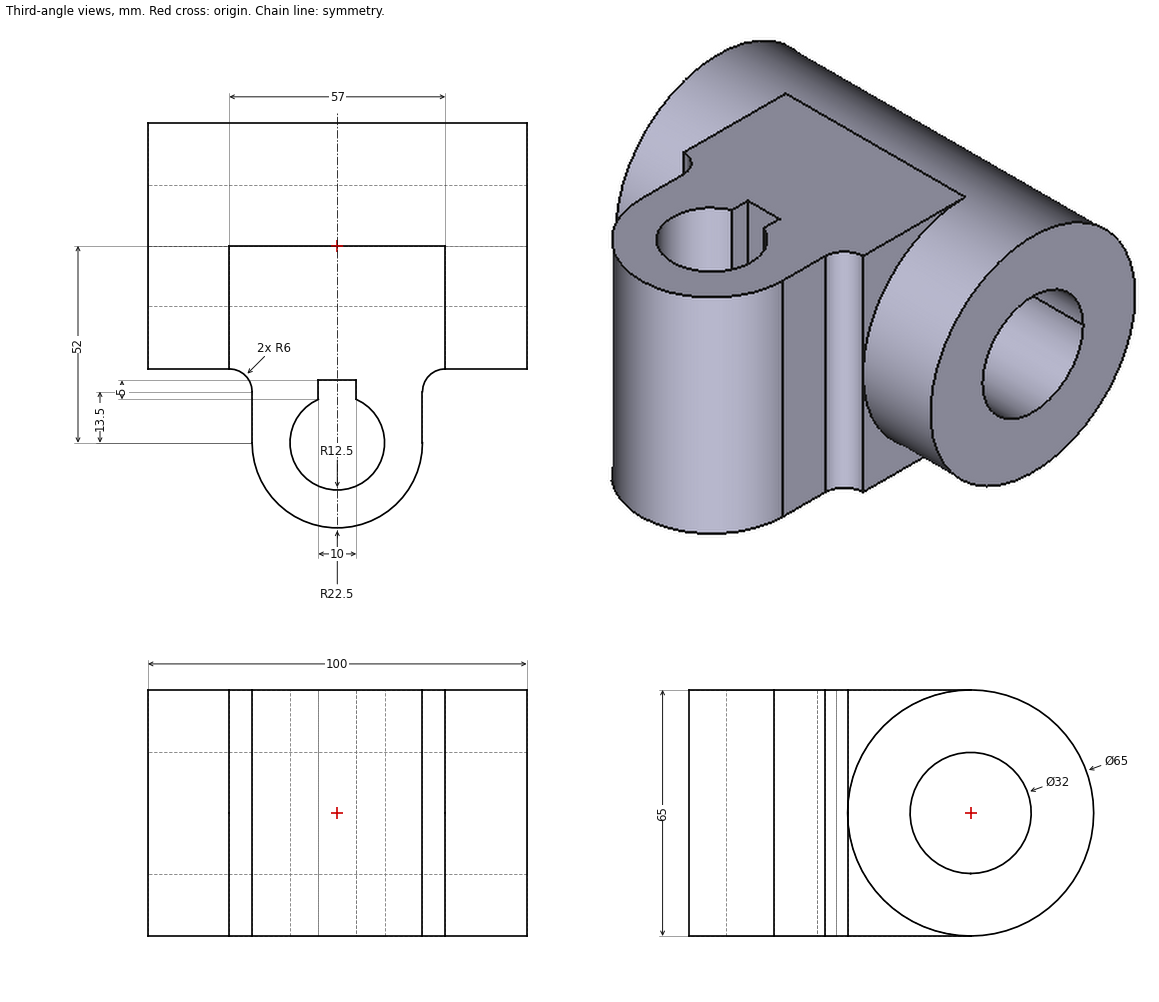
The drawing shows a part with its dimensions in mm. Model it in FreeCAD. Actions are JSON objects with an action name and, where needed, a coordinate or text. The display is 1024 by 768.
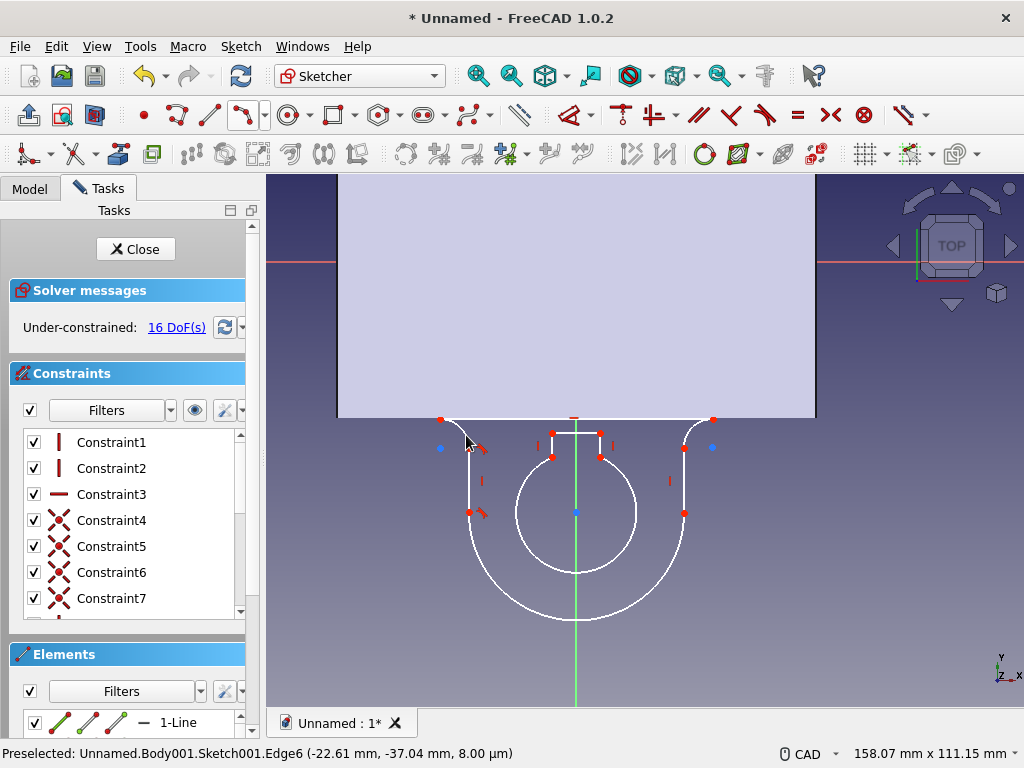
{"action": "left_click", "coordinate": [684, 494]}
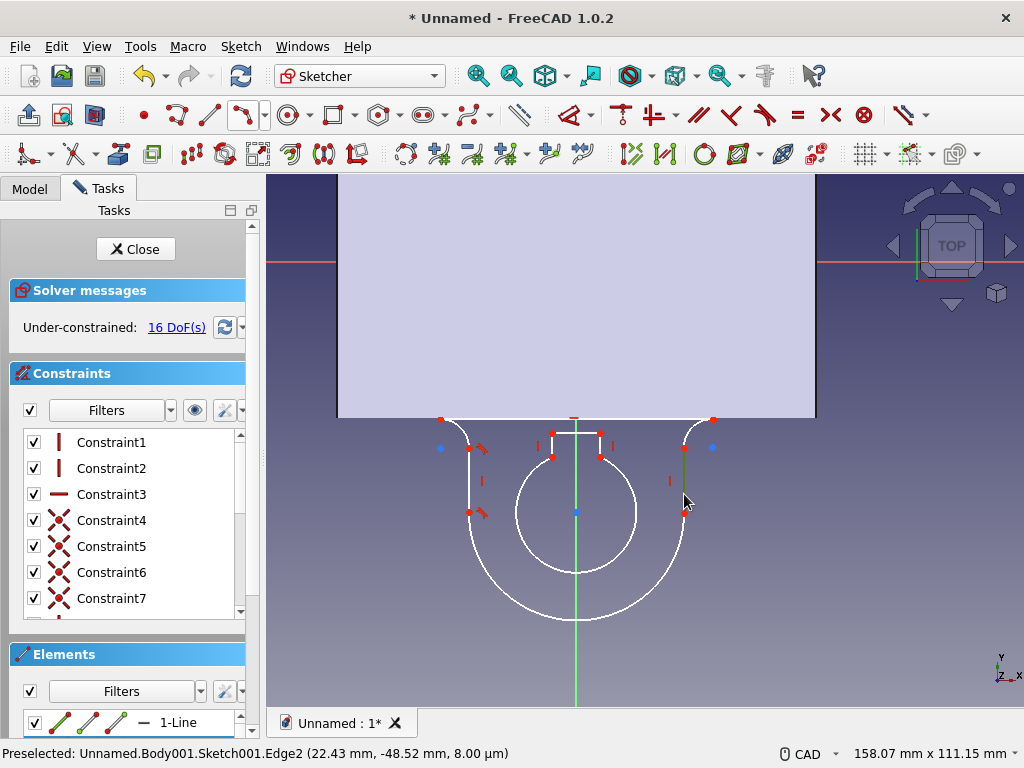
{"action": "left_click", "coordinate": [513, 600]}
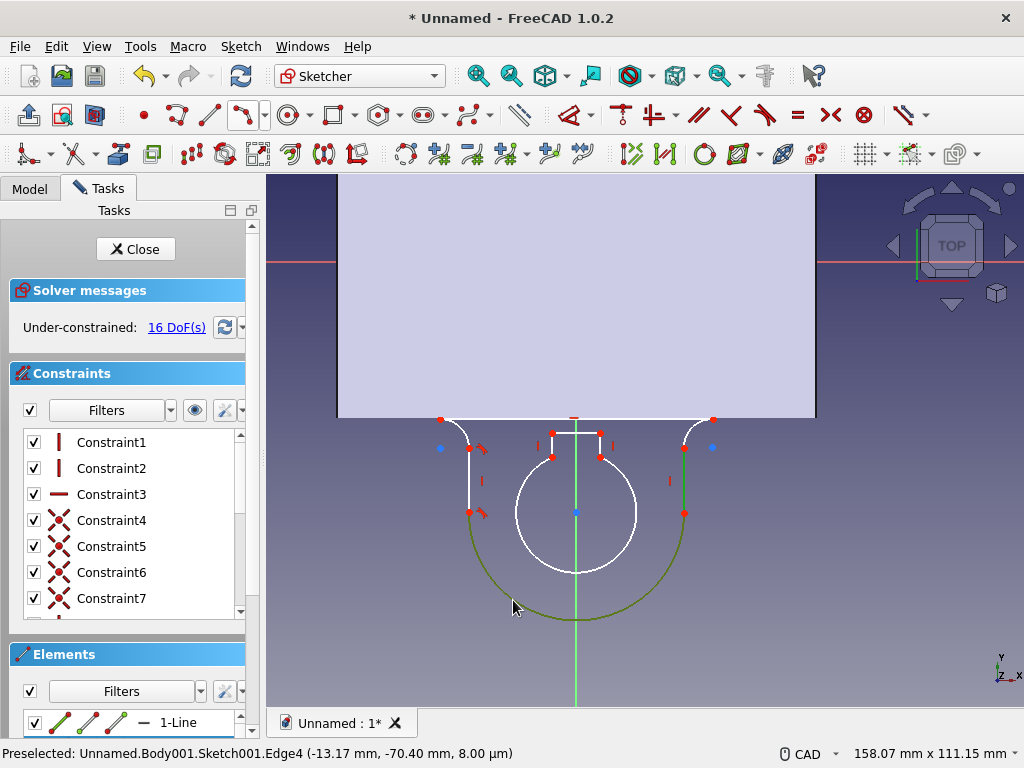
{"action": "key", "text": "t"}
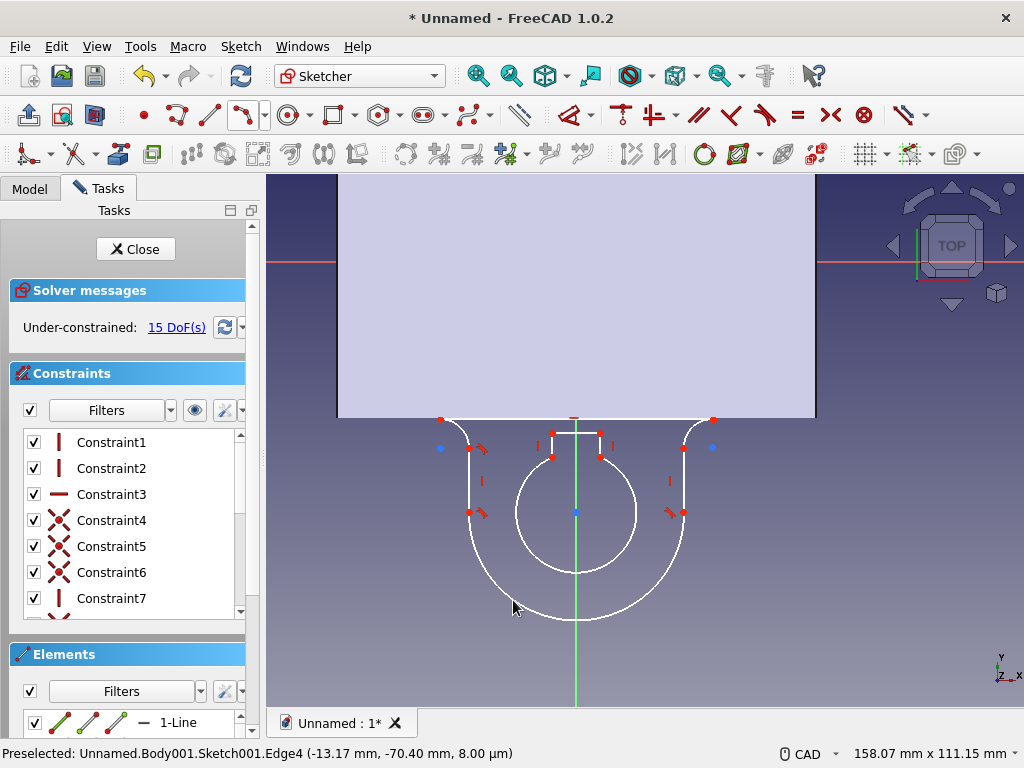
{"action": "left_click", "coordinate": [684, 494]}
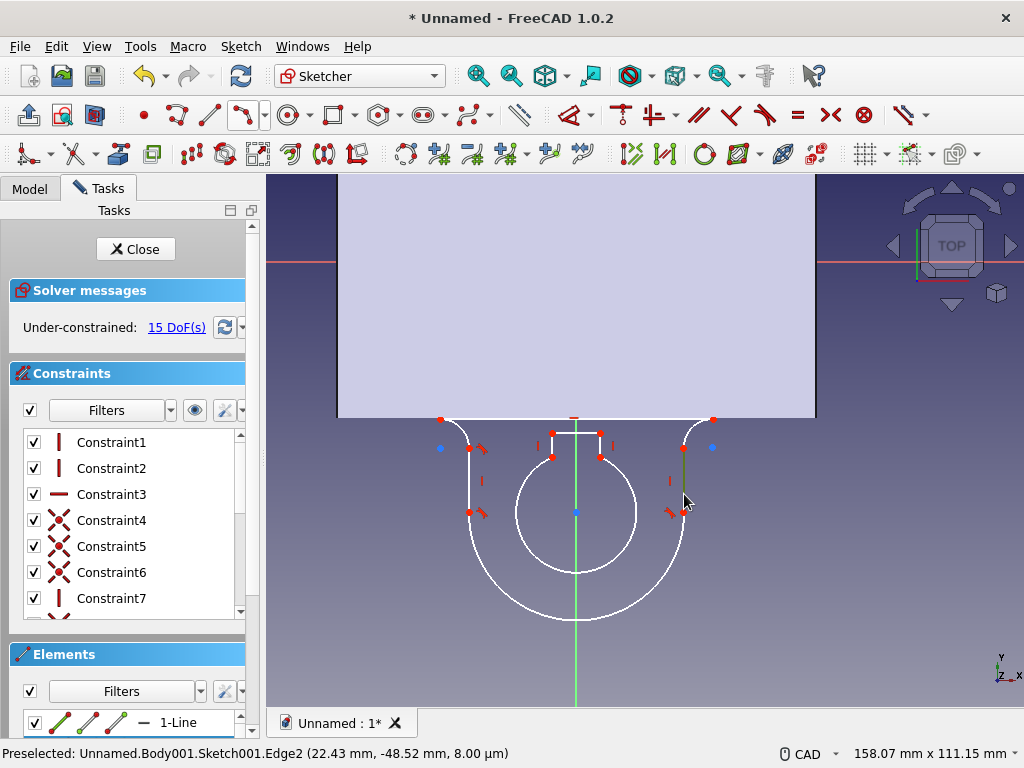
{"action": "left_click", "coordinate": [687, 435]}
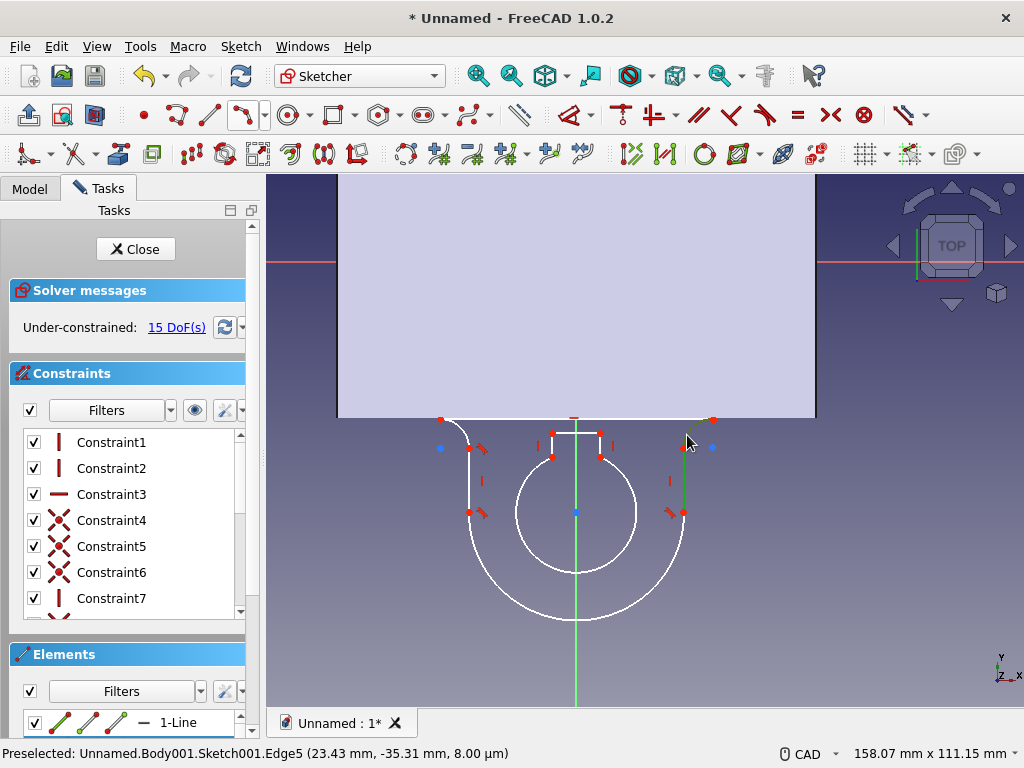
{"action": "key", "text": "t"}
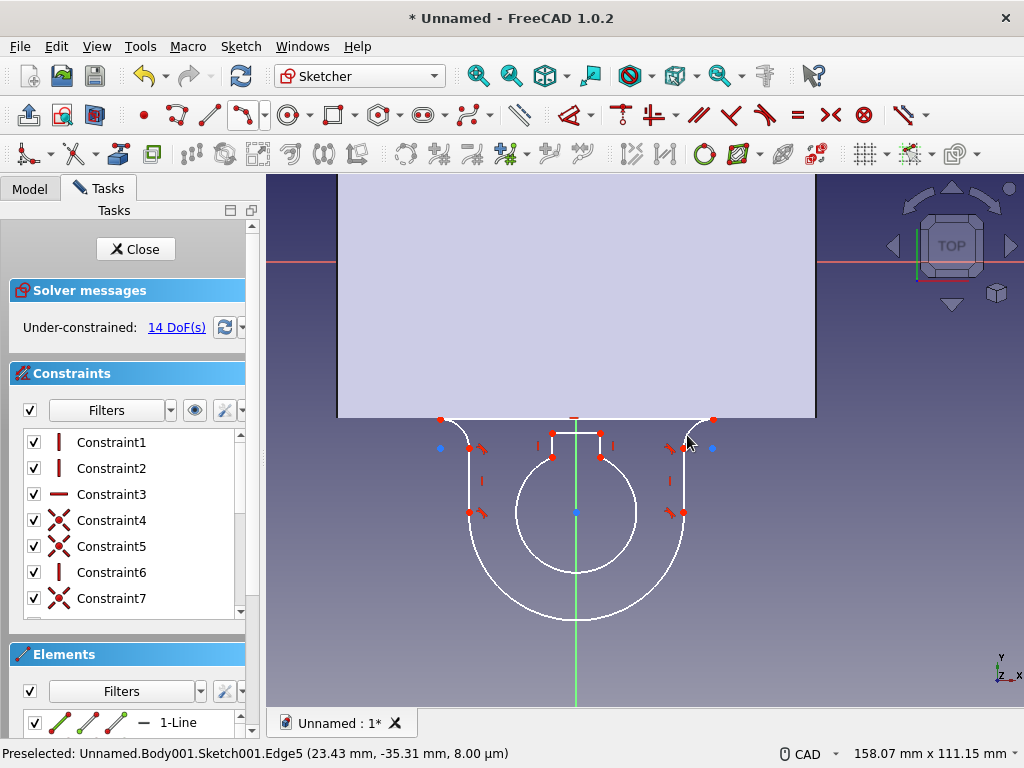
{"action": "left_click", "coordinate": [631, 419]}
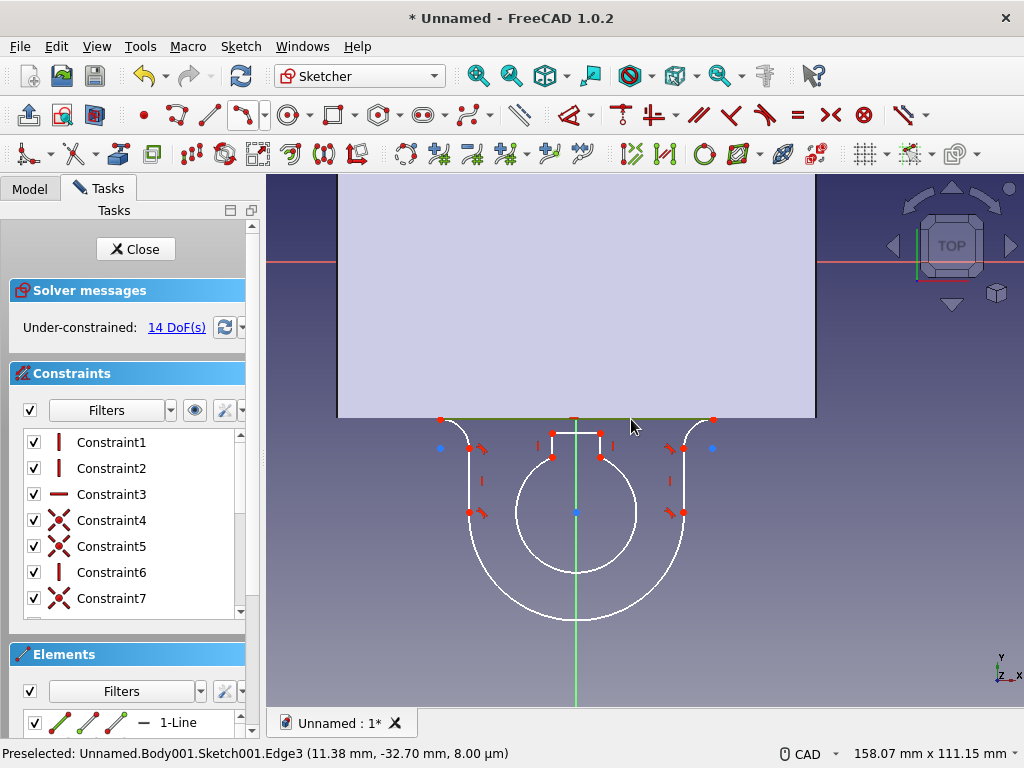
{"action": "left_click", "coordinate": [687, 435]}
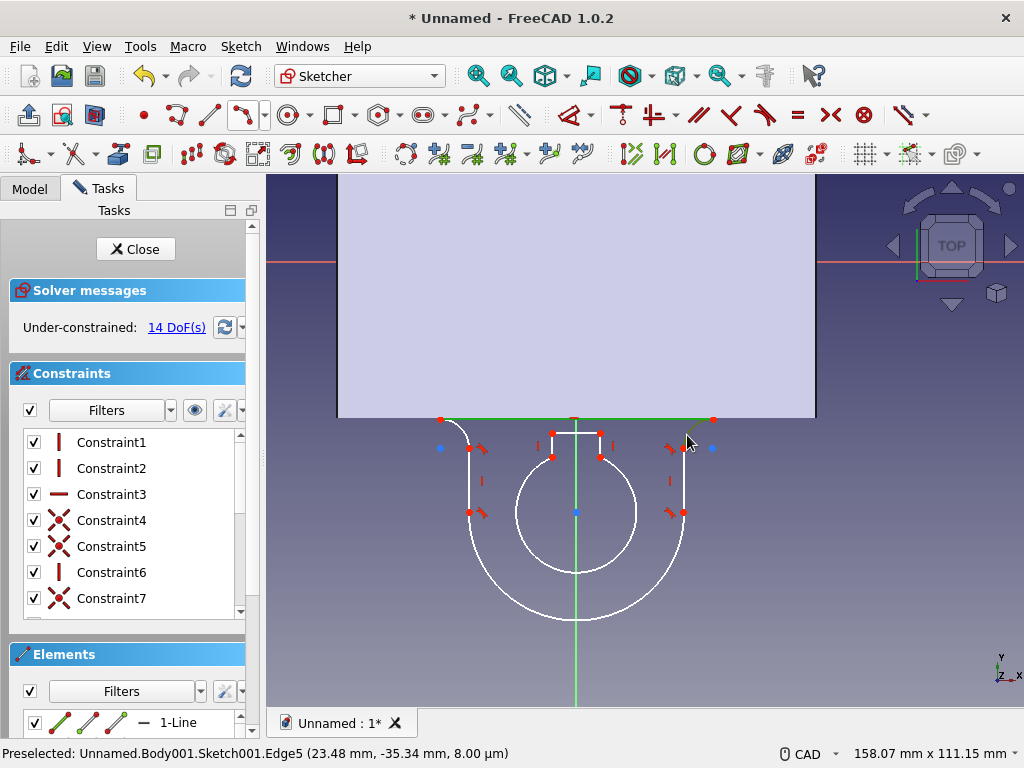
{"action": "left_click", "coordinate": [765, 116]}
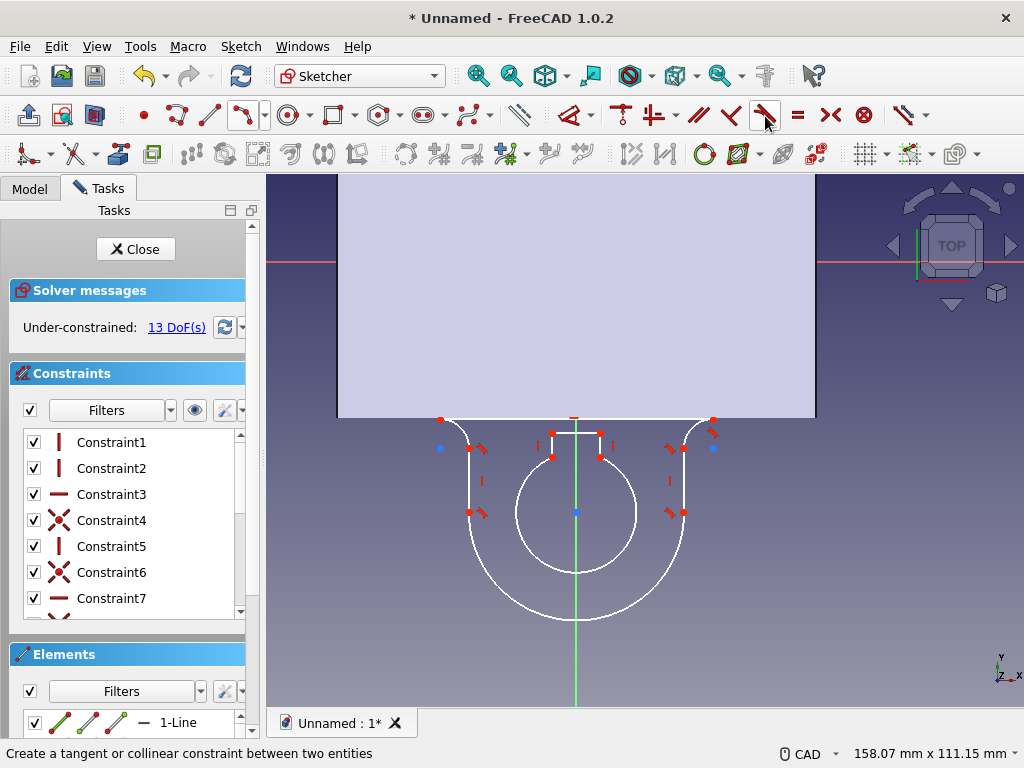
{"action": "left_click", "coordinate": [631, 419]}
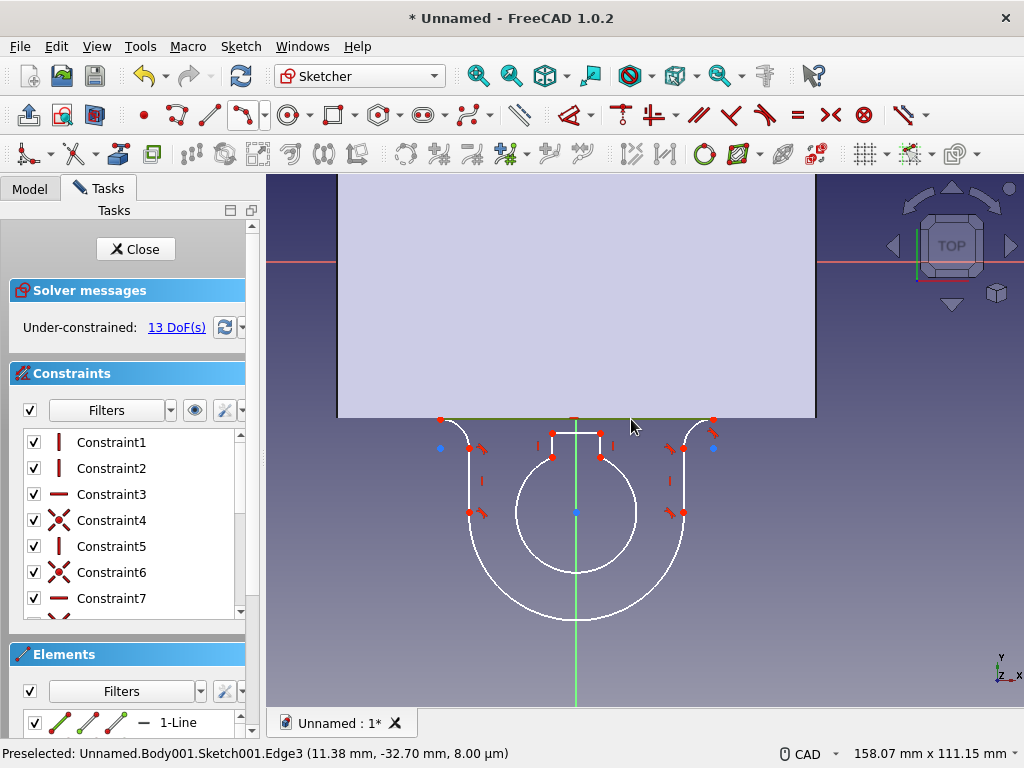
{"action": "left_click", "coordinate": [466, 435]}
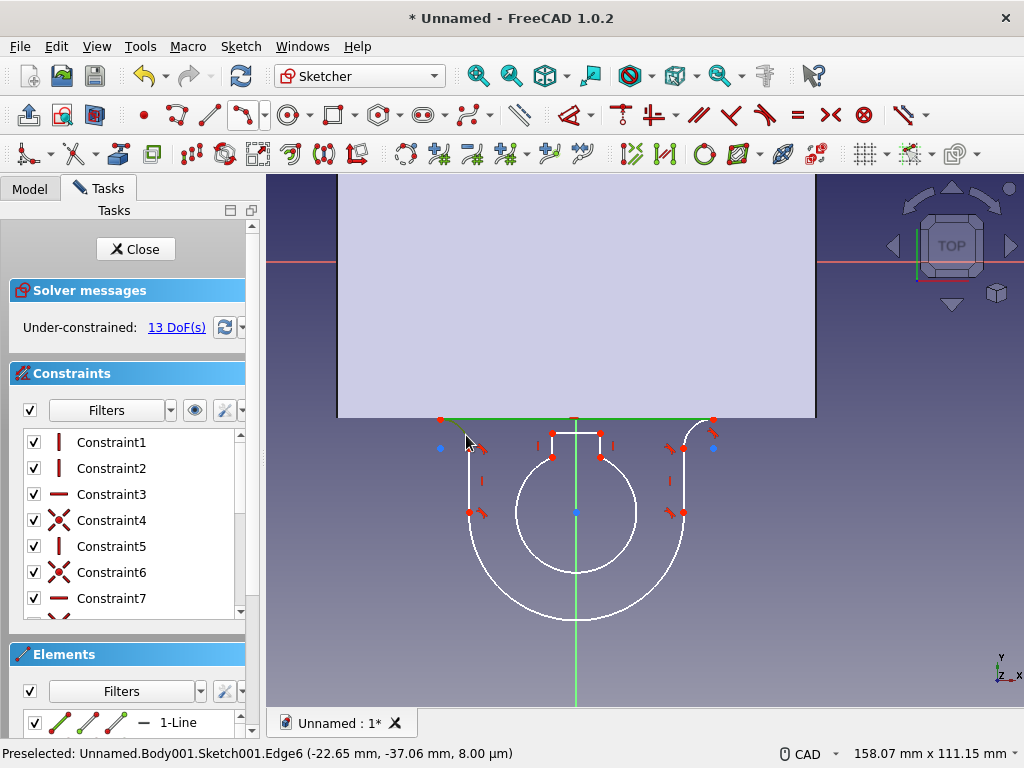
{"action": "key", "text": "t"}